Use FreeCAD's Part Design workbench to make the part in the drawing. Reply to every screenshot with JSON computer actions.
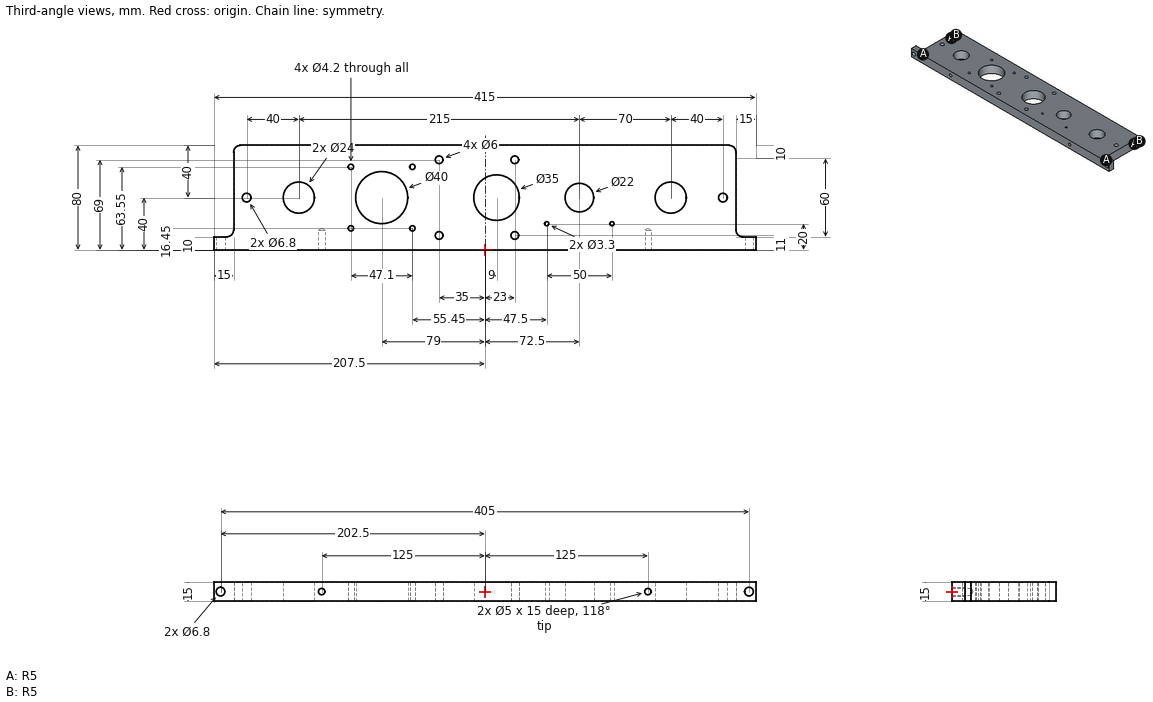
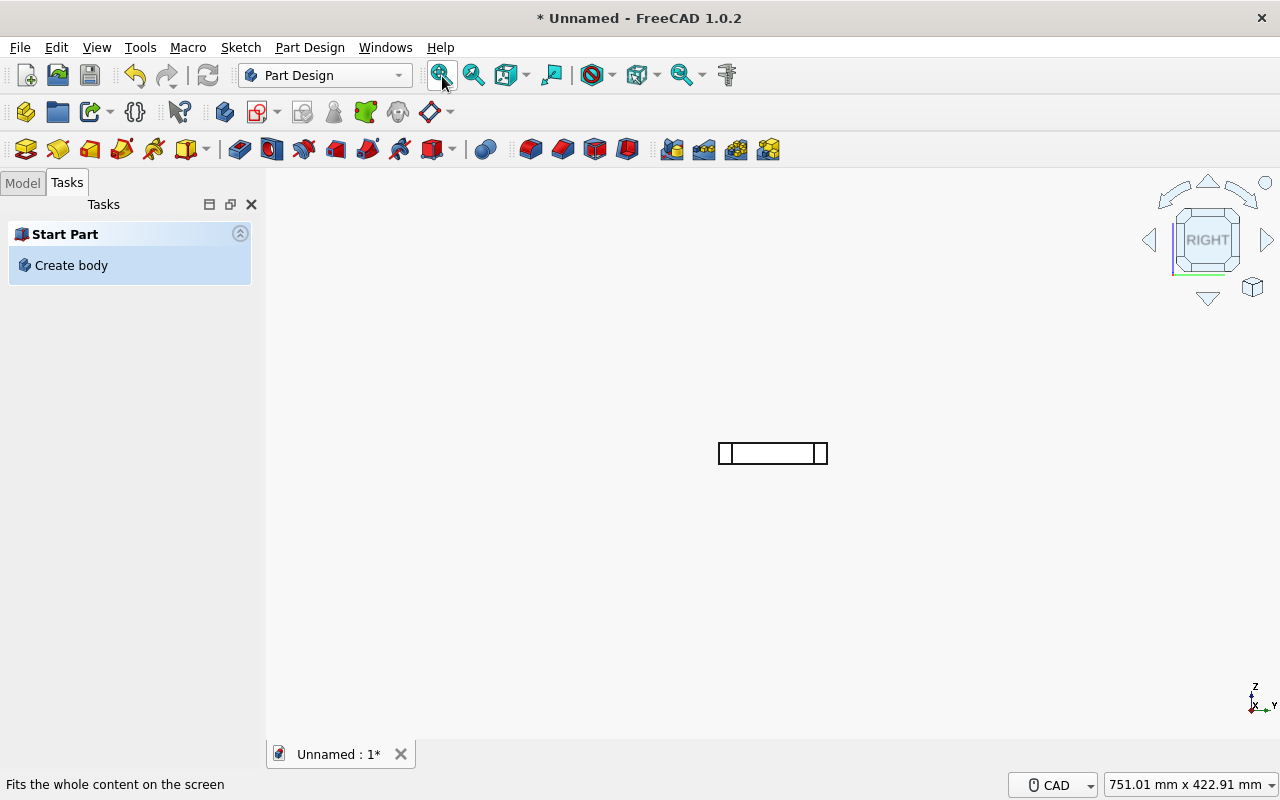
{"action": "left_click", "coordinate": [442, 76]}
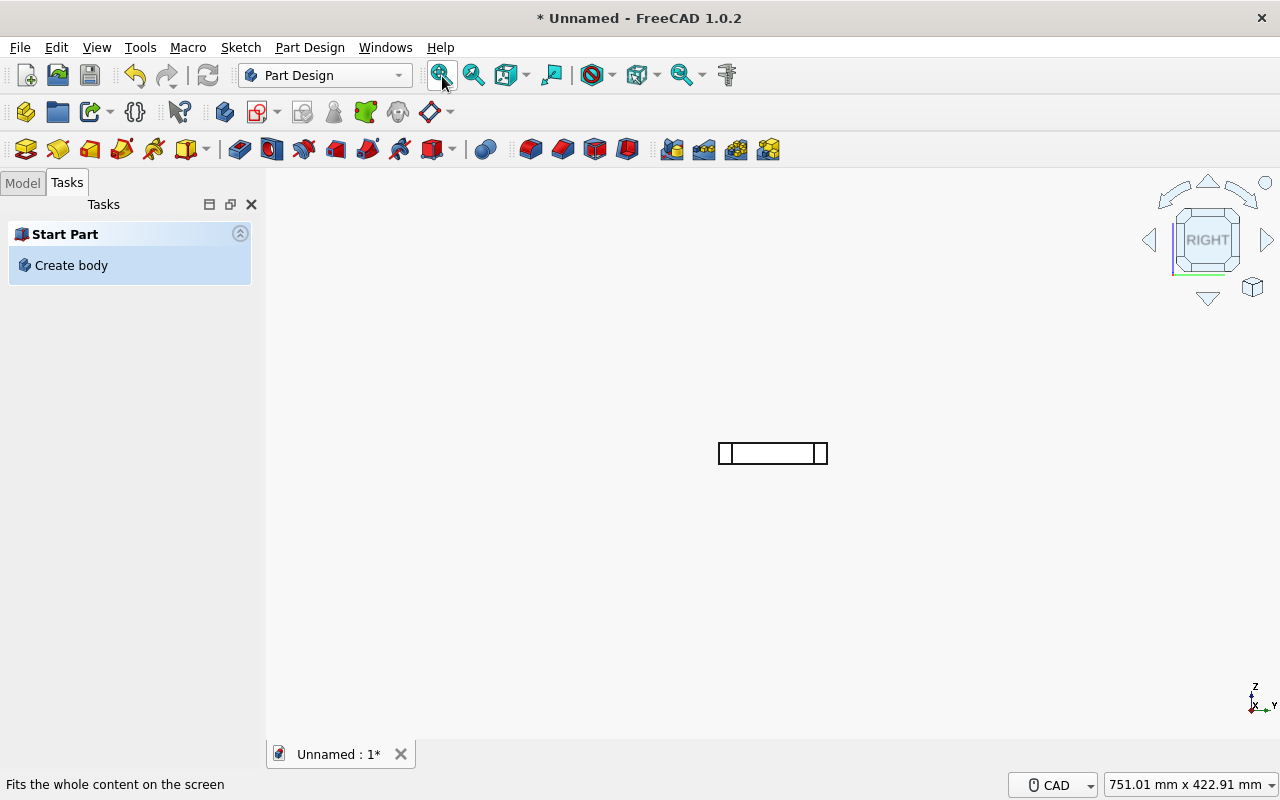
{"action": "scroll", "coordinate": [732, 452], "scroll_direction": "up", "scroll_amount": 4}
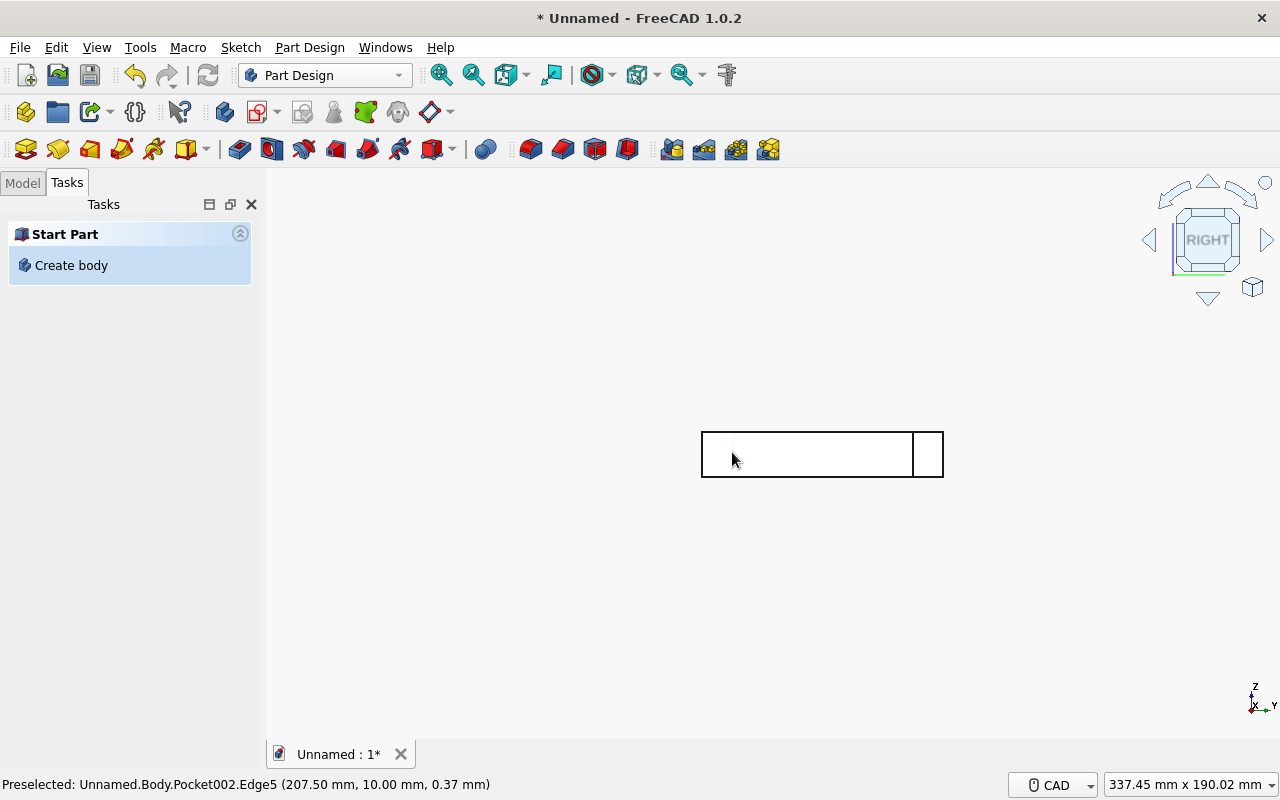
{"action": "left_click", "coordinate": [442, 76]}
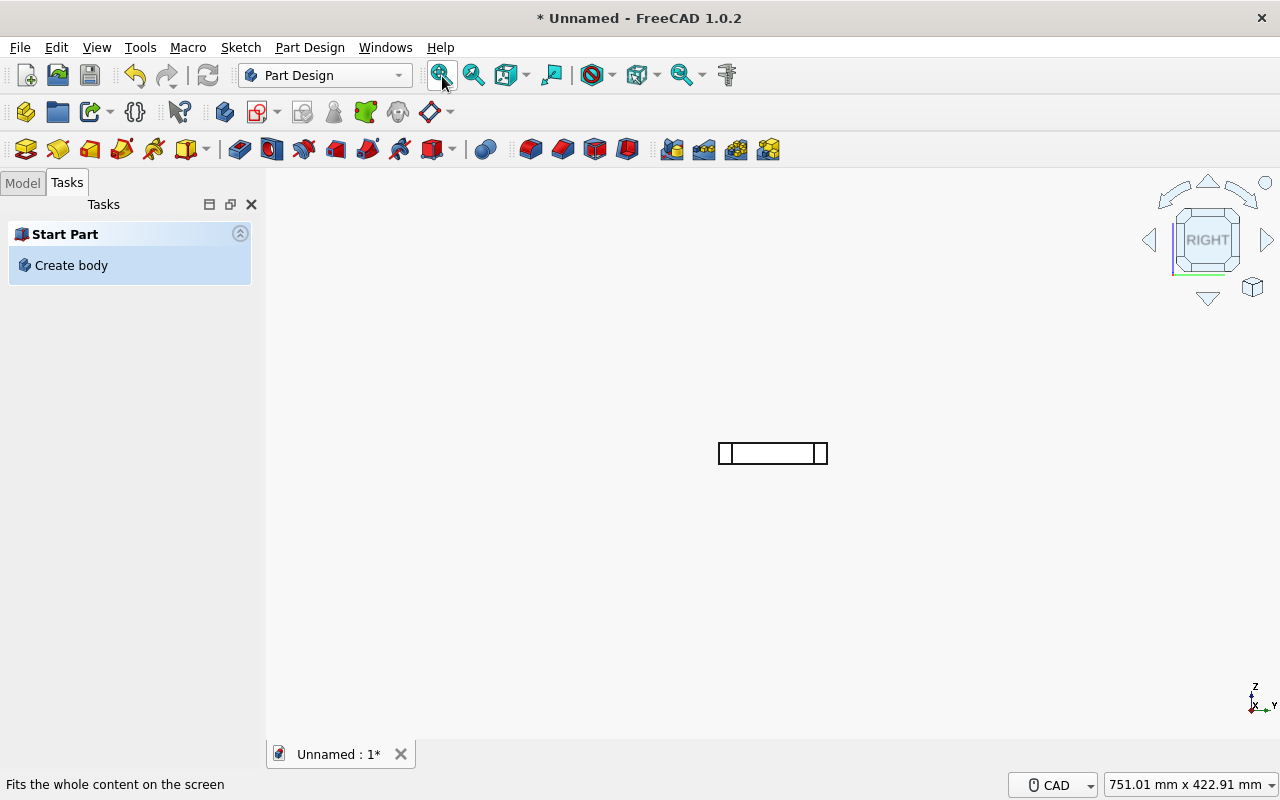
{"action": "key", "text": "5"}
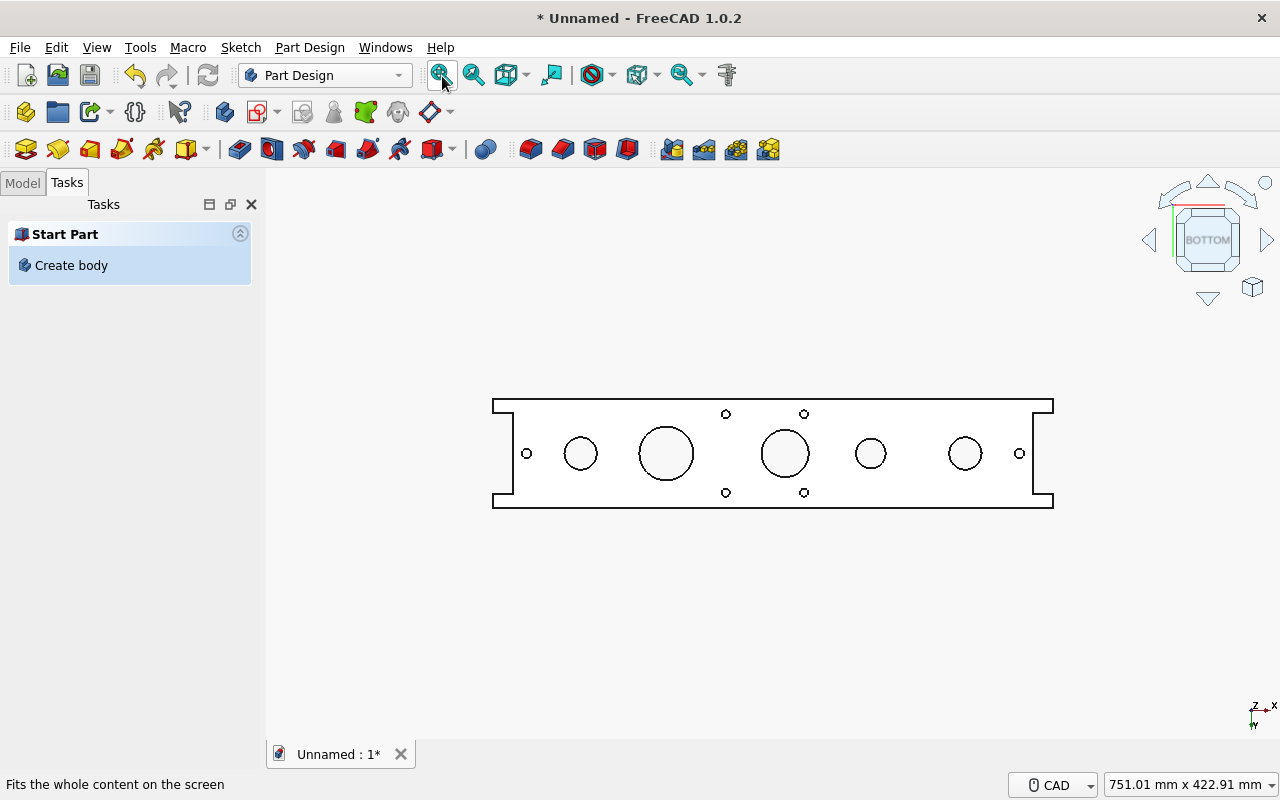
{"action": "scroll", "coordinate": [513, 412], "scroll_direction": "up", "scroll_amount": 4}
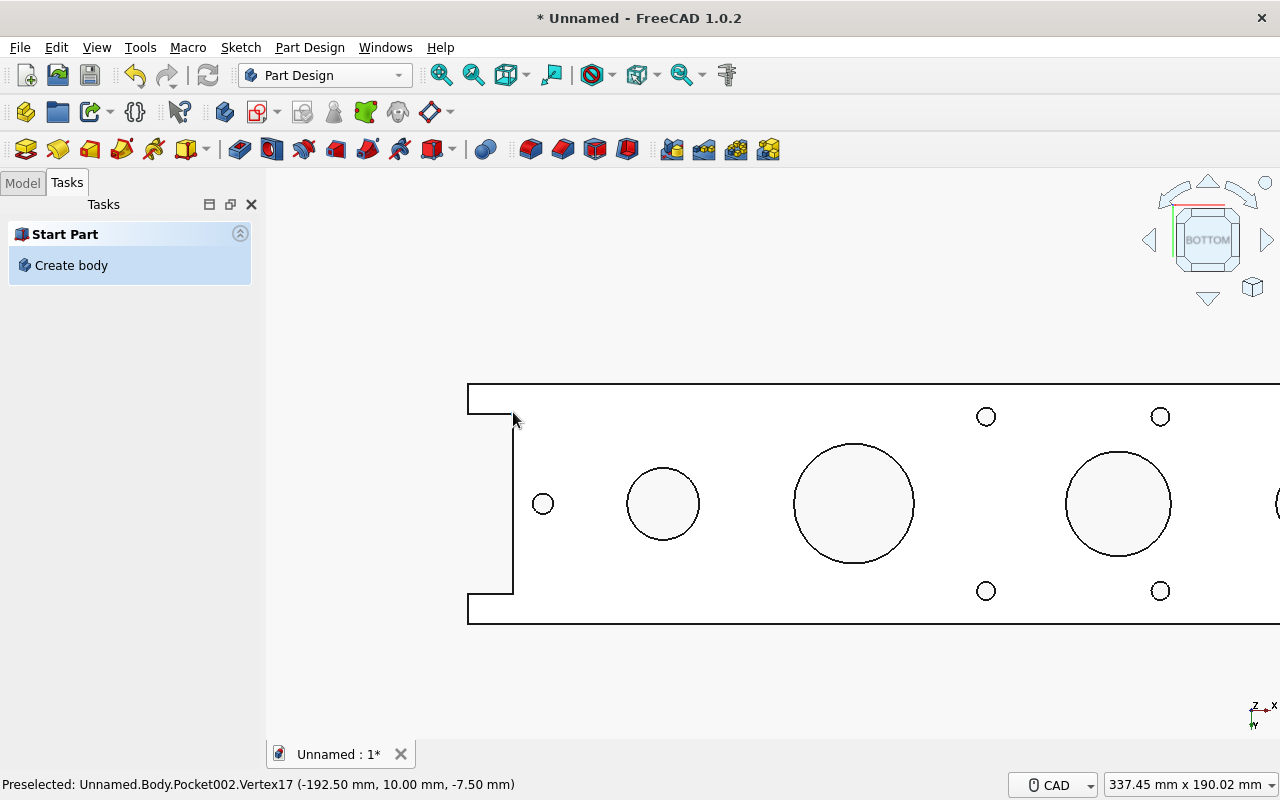
{"action": "left_click", "coordinate": [442, 76]}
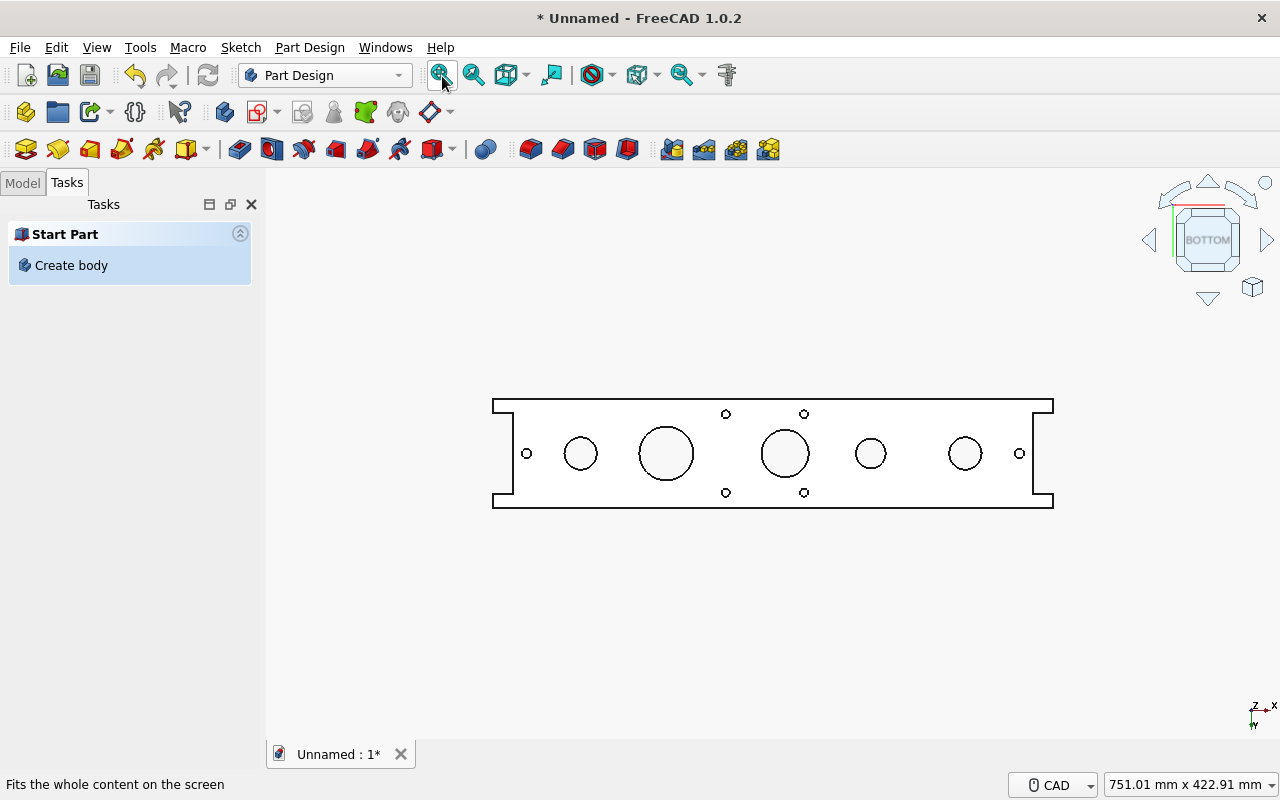
{"action": "key", "text": "4"}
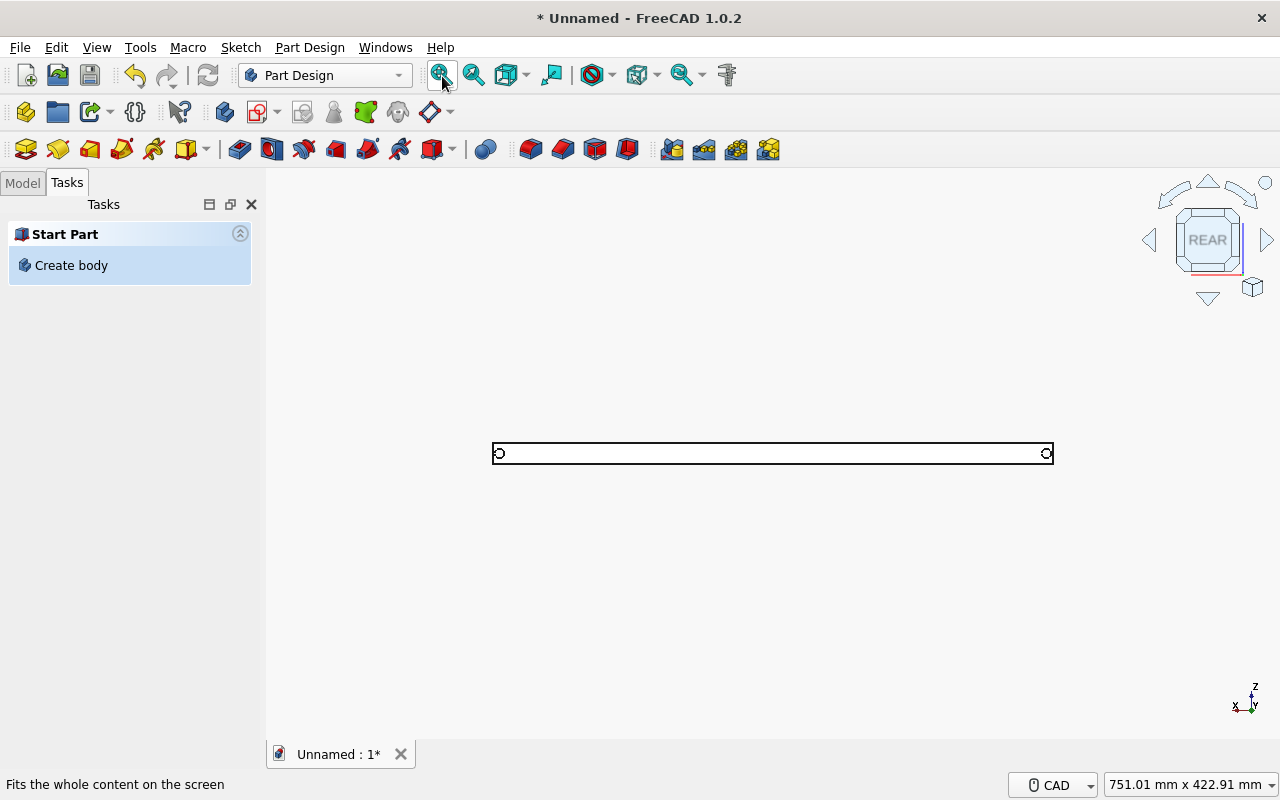
{"action": "scroll", "coordinate": [1033, 452], "scroll_direction": "up", "scroll_amount": 4}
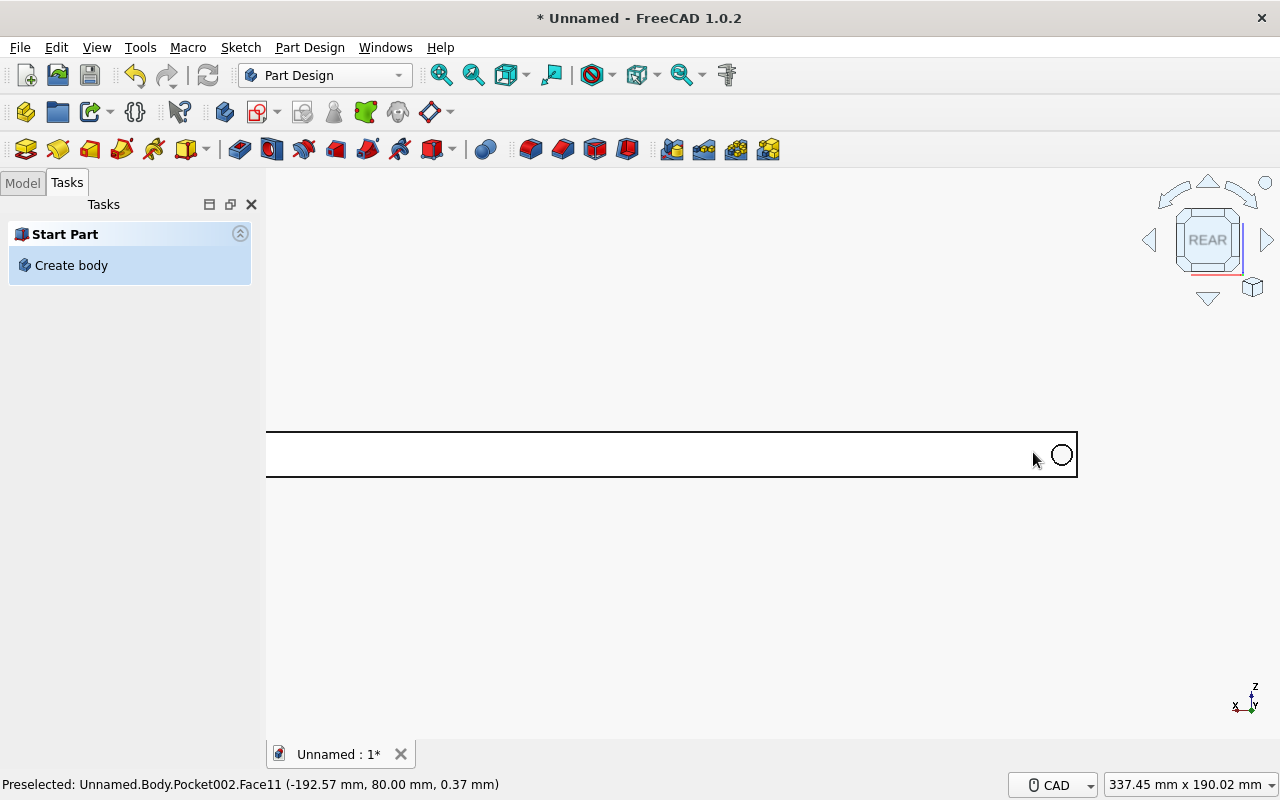
{"action": "left_click", "coordinate": [442, 76]}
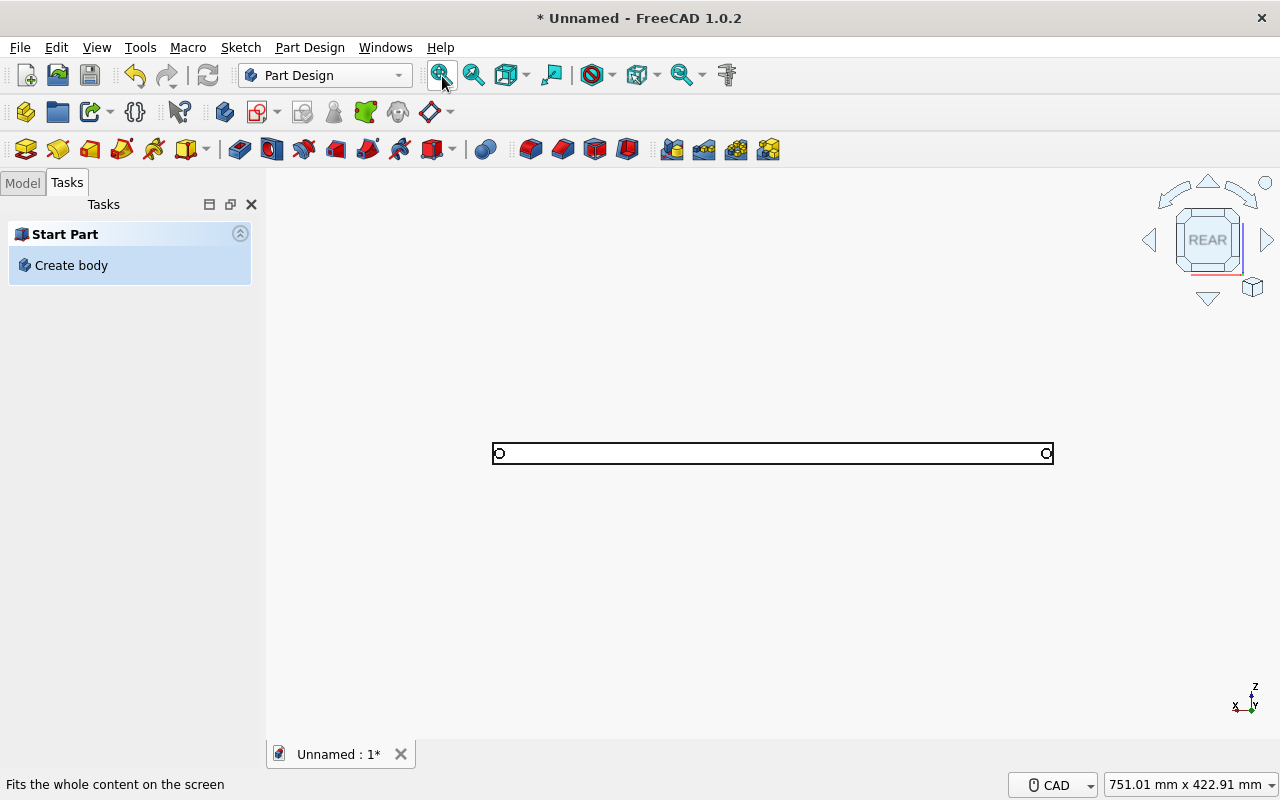
{"action": "key", "text": "6"}